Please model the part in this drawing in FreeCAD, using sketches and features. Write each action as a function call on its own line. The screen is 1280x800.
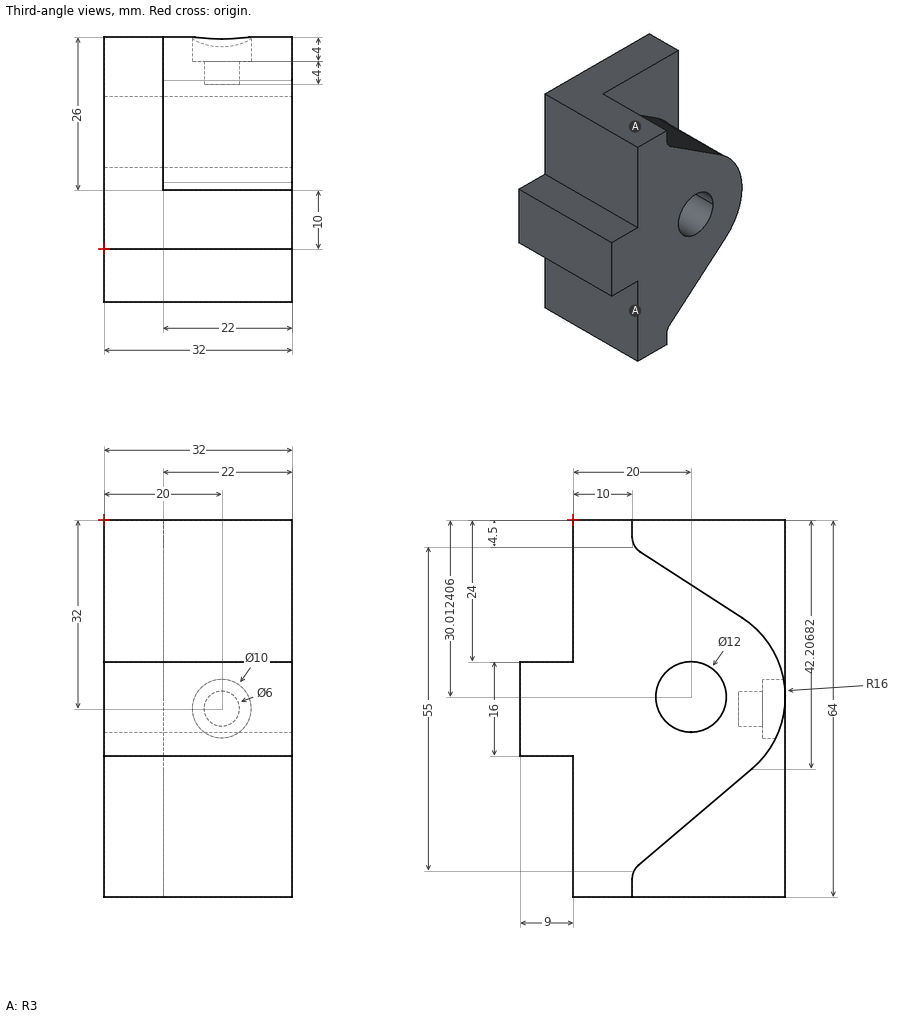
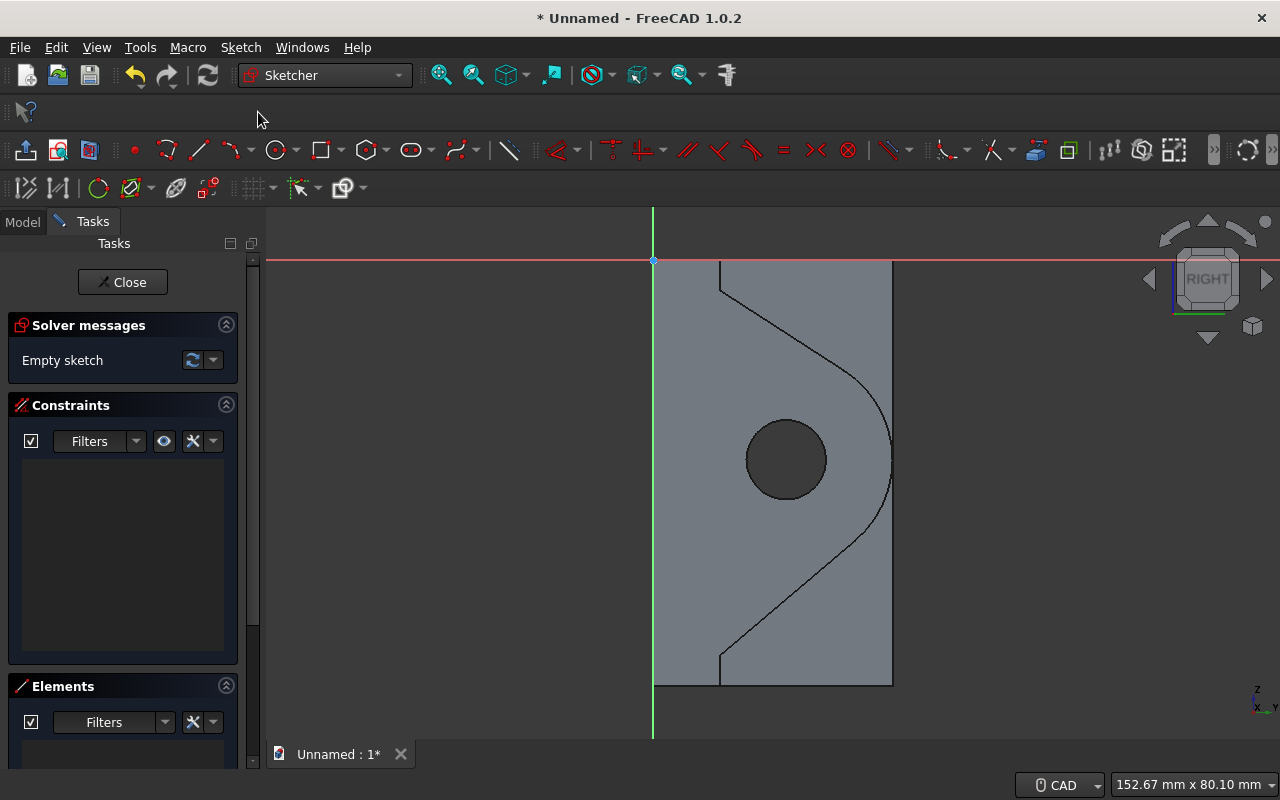
scroll(589, 473, up, 6)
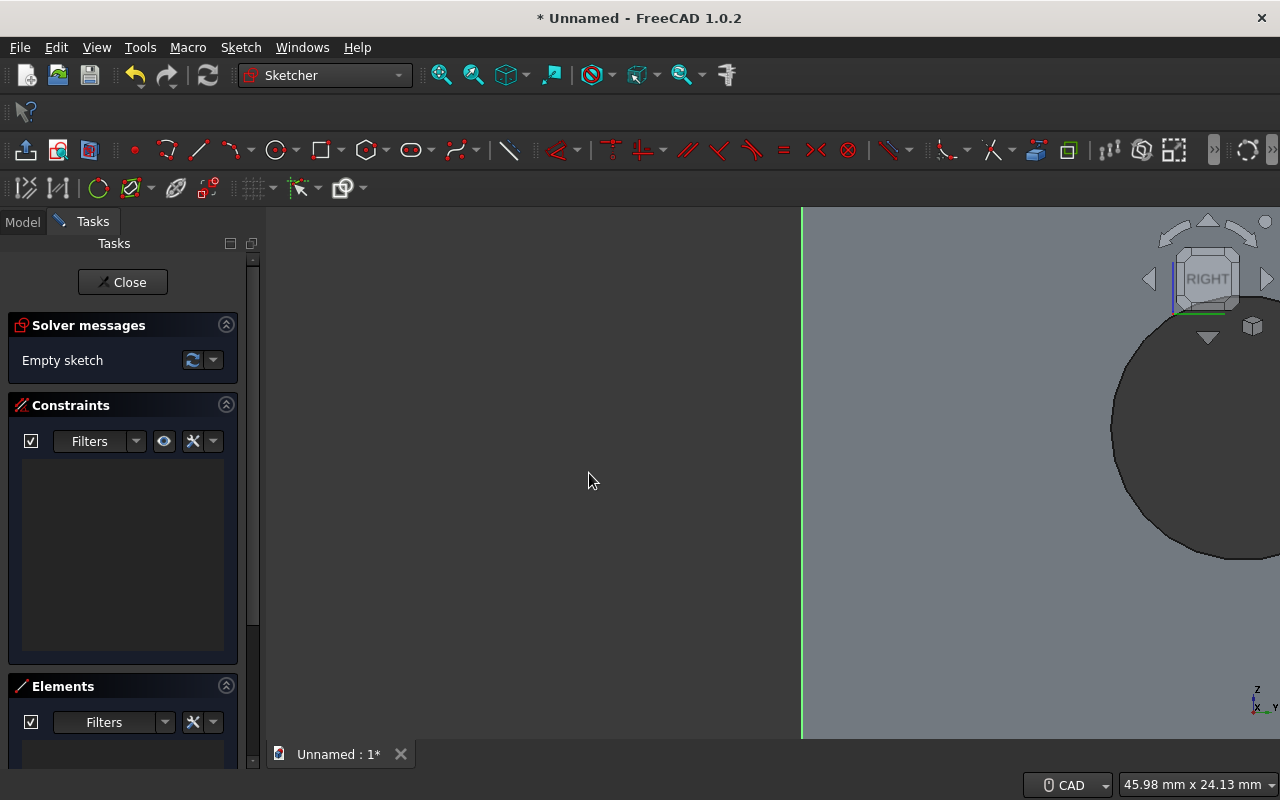
key(g)
key(r)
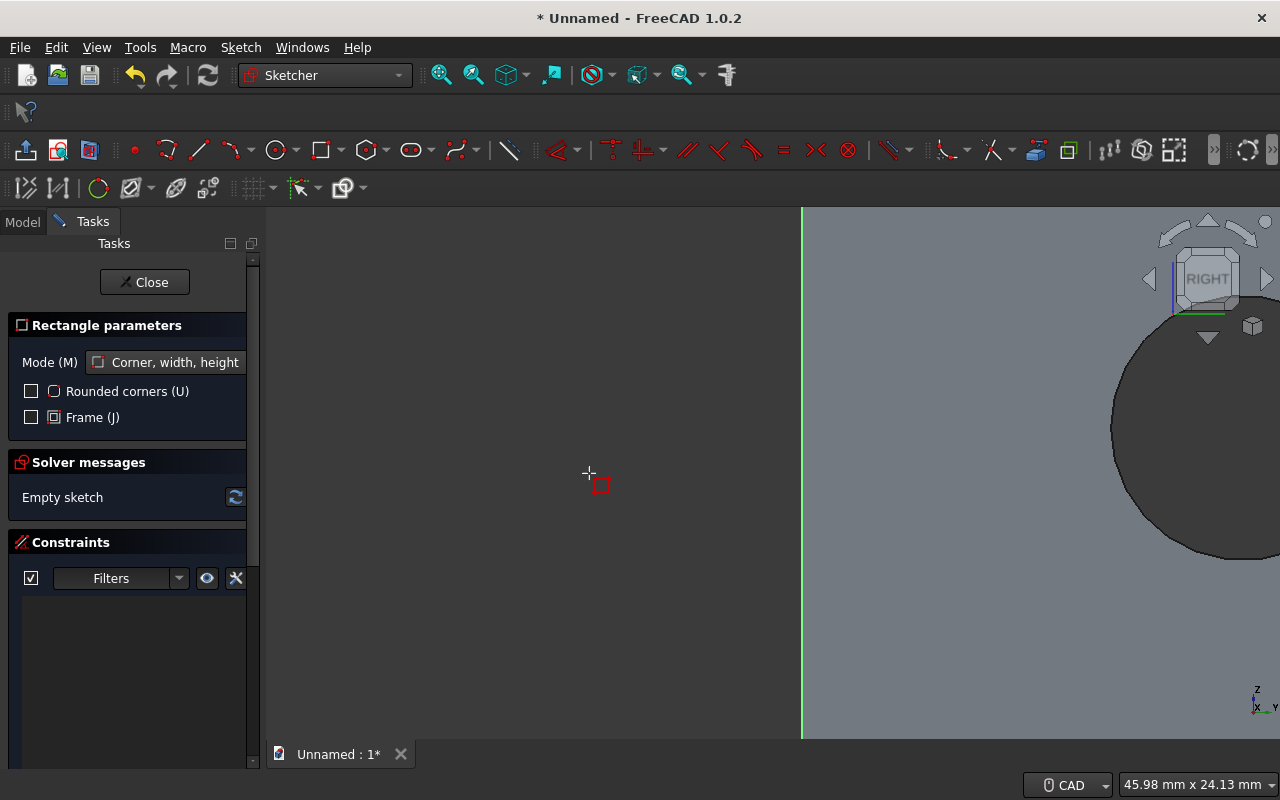
click(604, 295)
click(802, 648)
key(Escape)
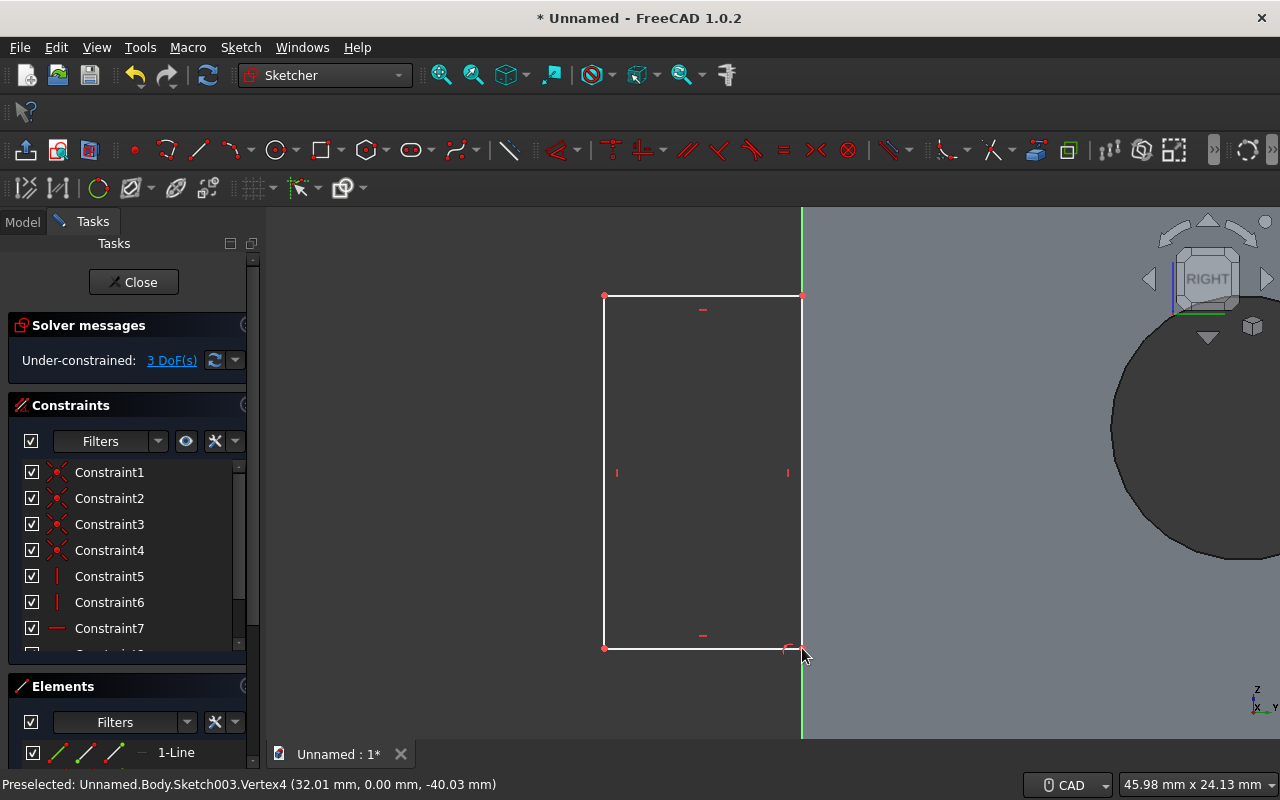
key(d)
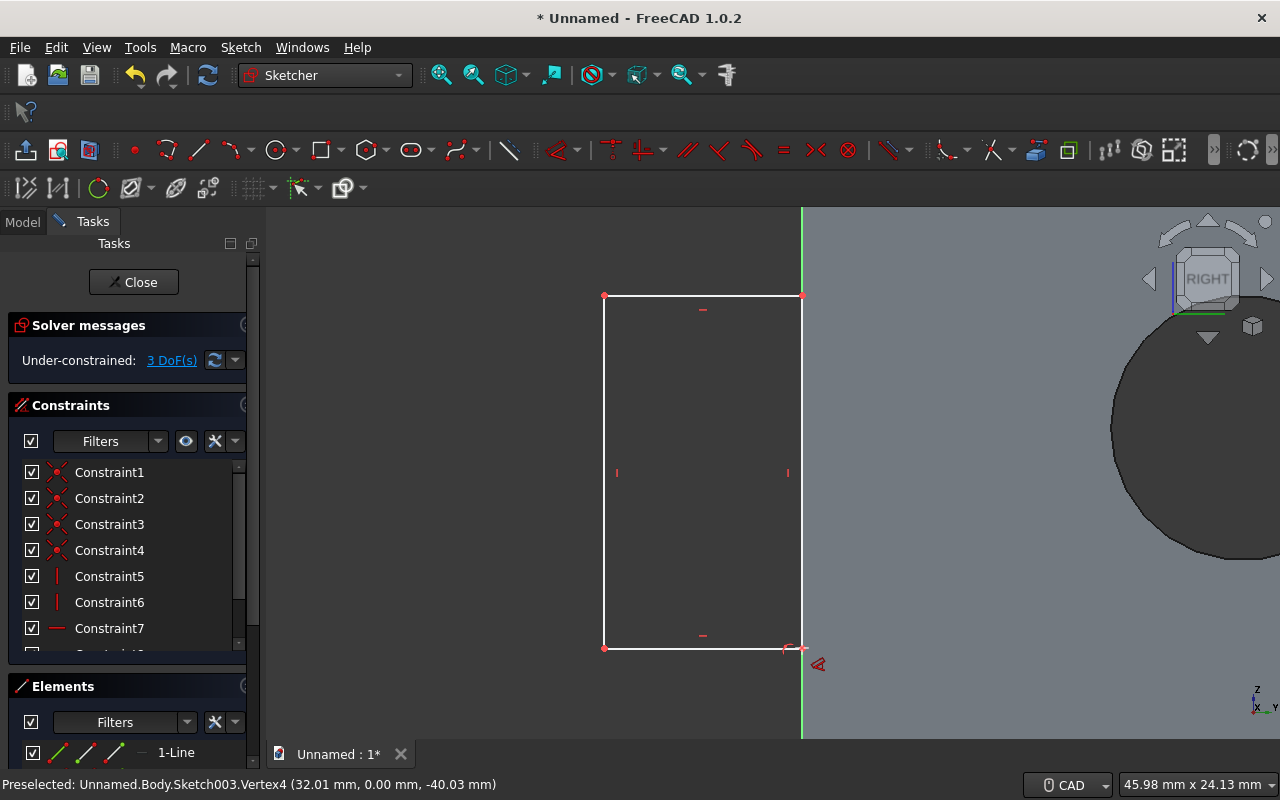
click(663, 649)
click(703, 683)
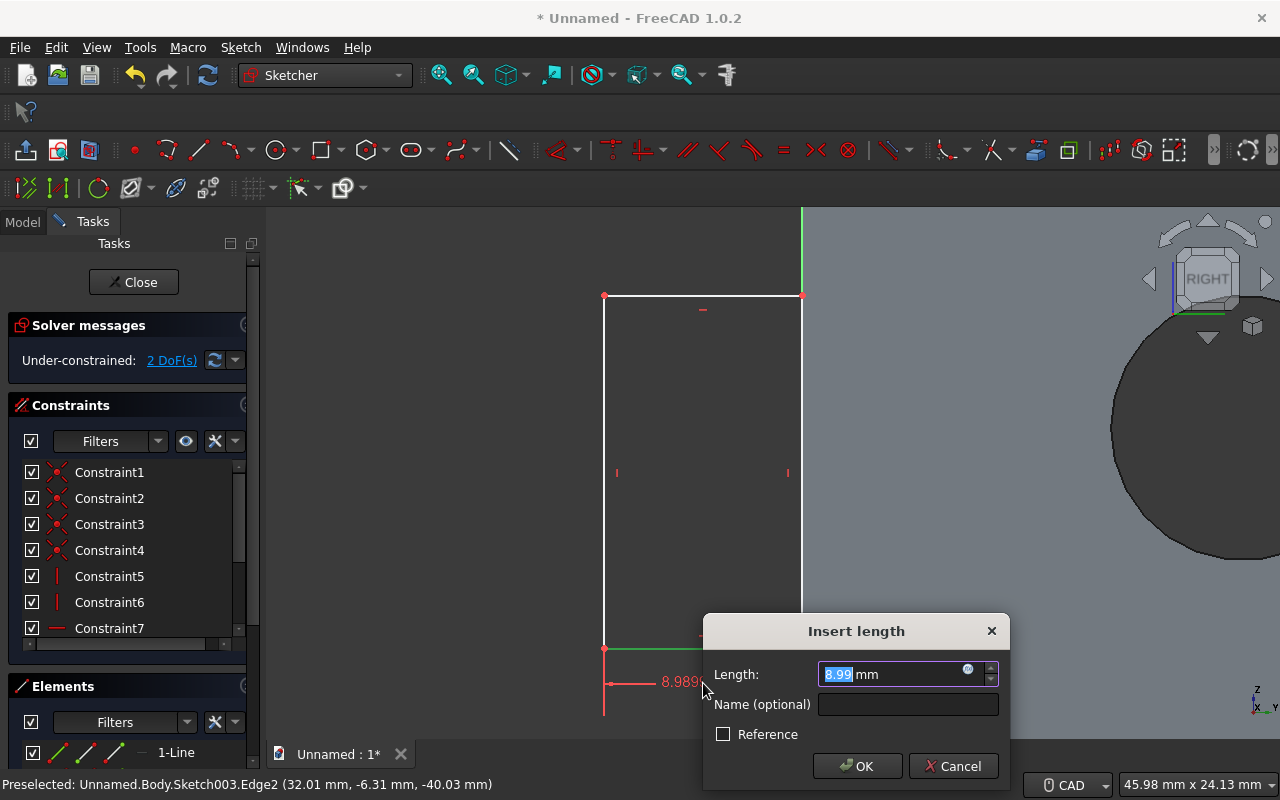
text(9)
key(Return)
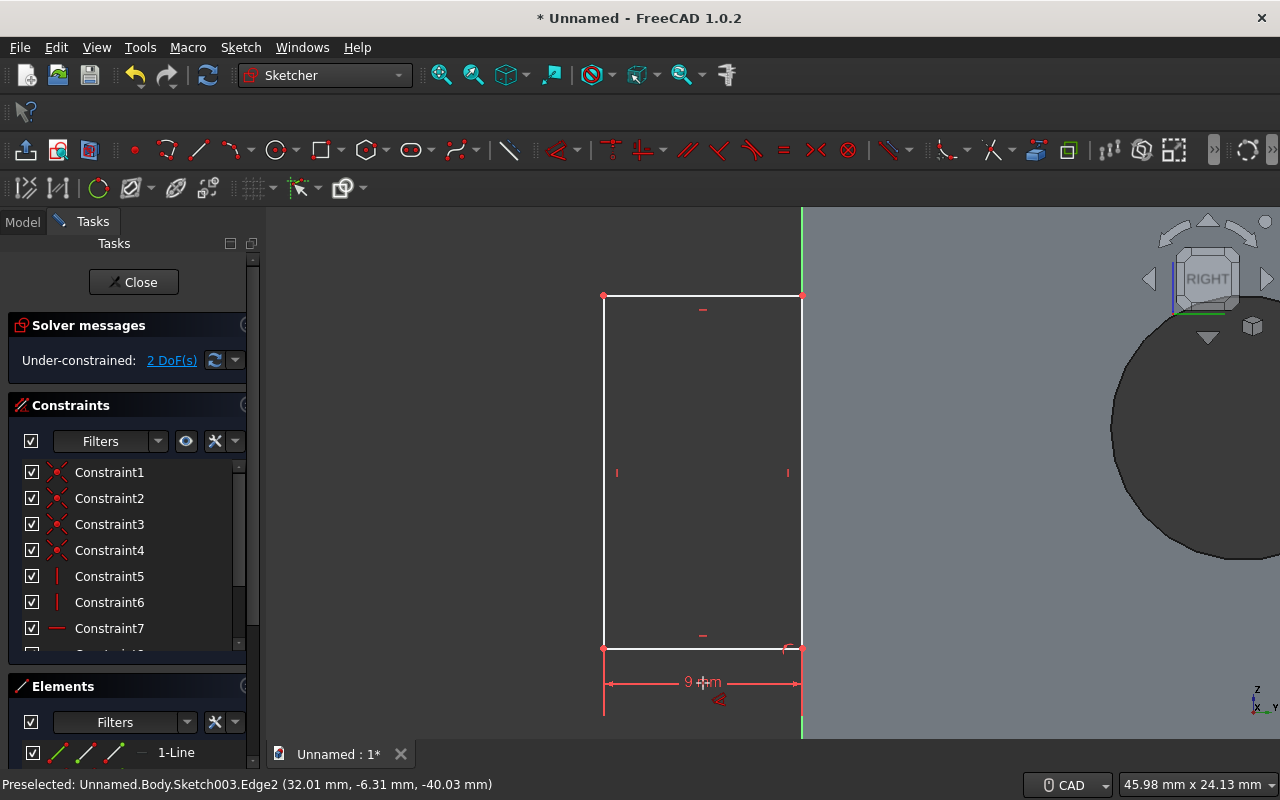
click(604, 402)
click(570, 472)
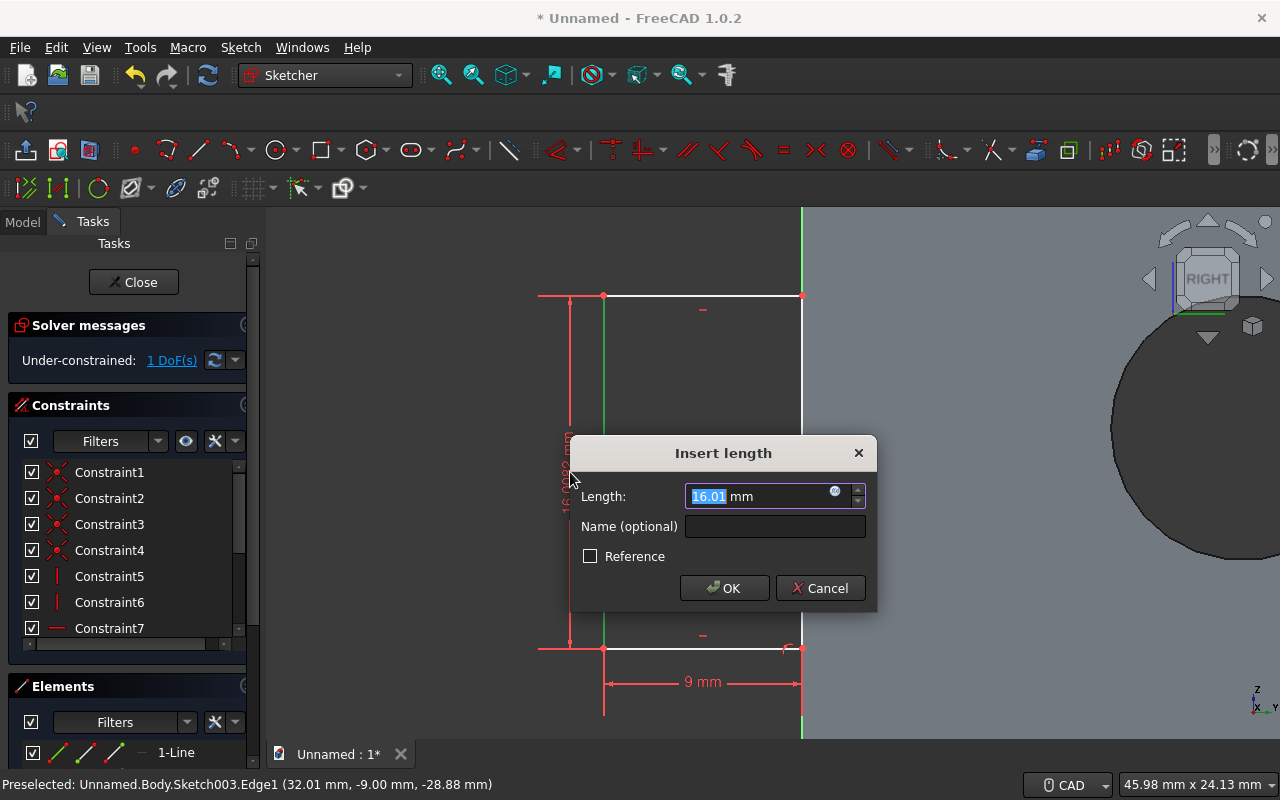
text(16)
key(Return)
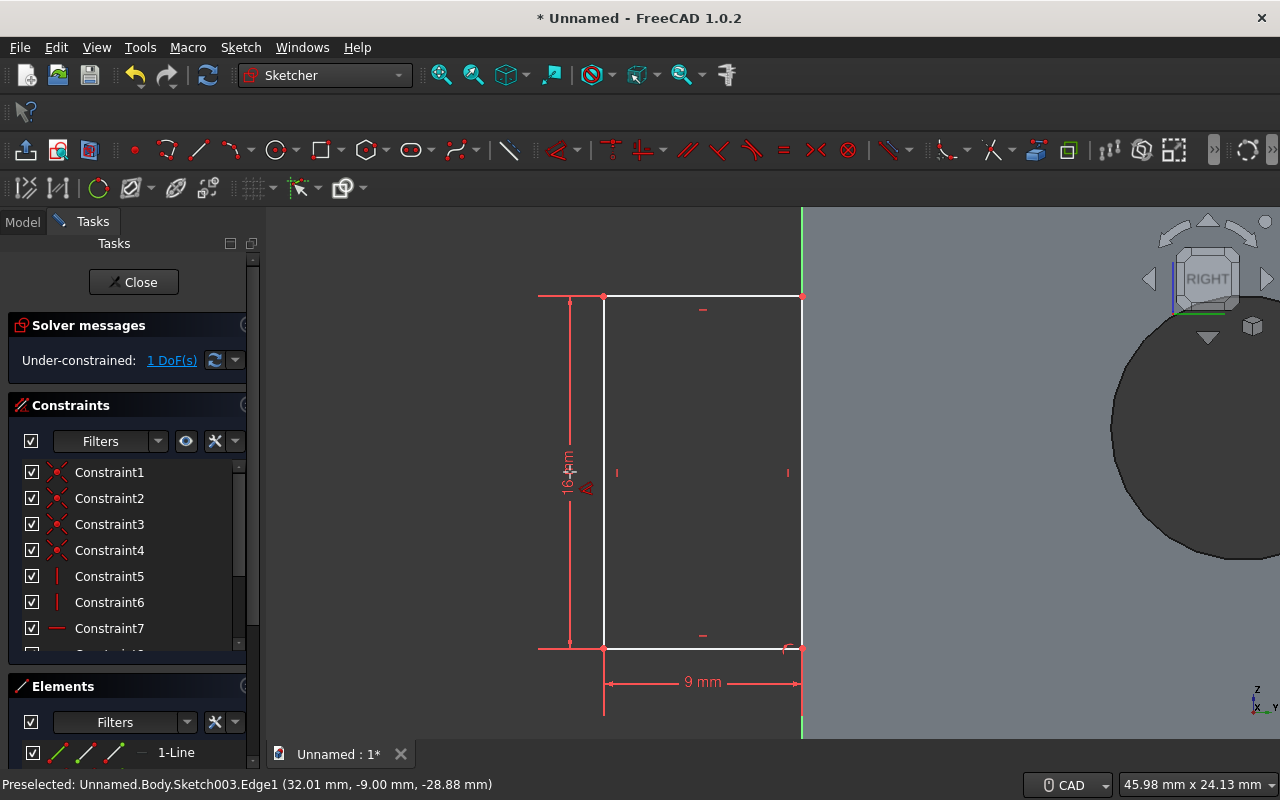
click(604, 296)
click(836, 266)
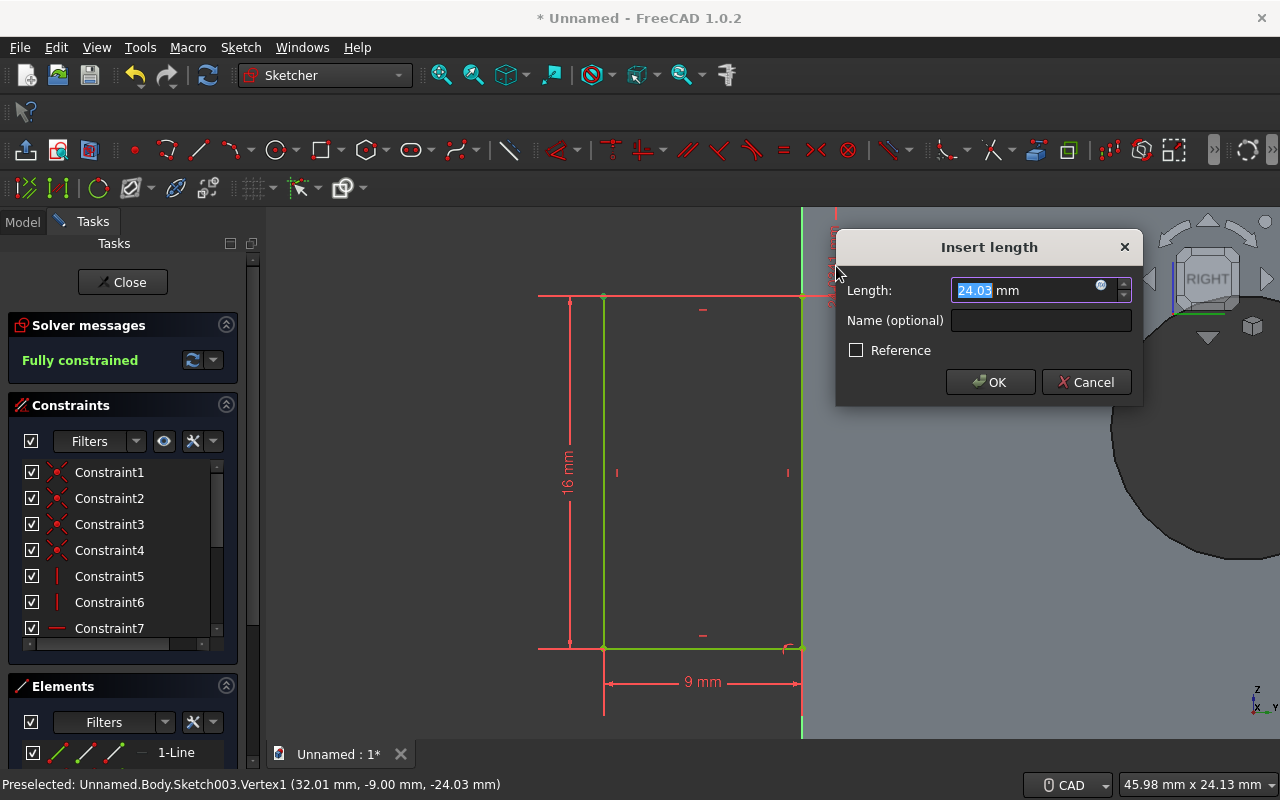
text(24)
key(Return)
key(Escape)